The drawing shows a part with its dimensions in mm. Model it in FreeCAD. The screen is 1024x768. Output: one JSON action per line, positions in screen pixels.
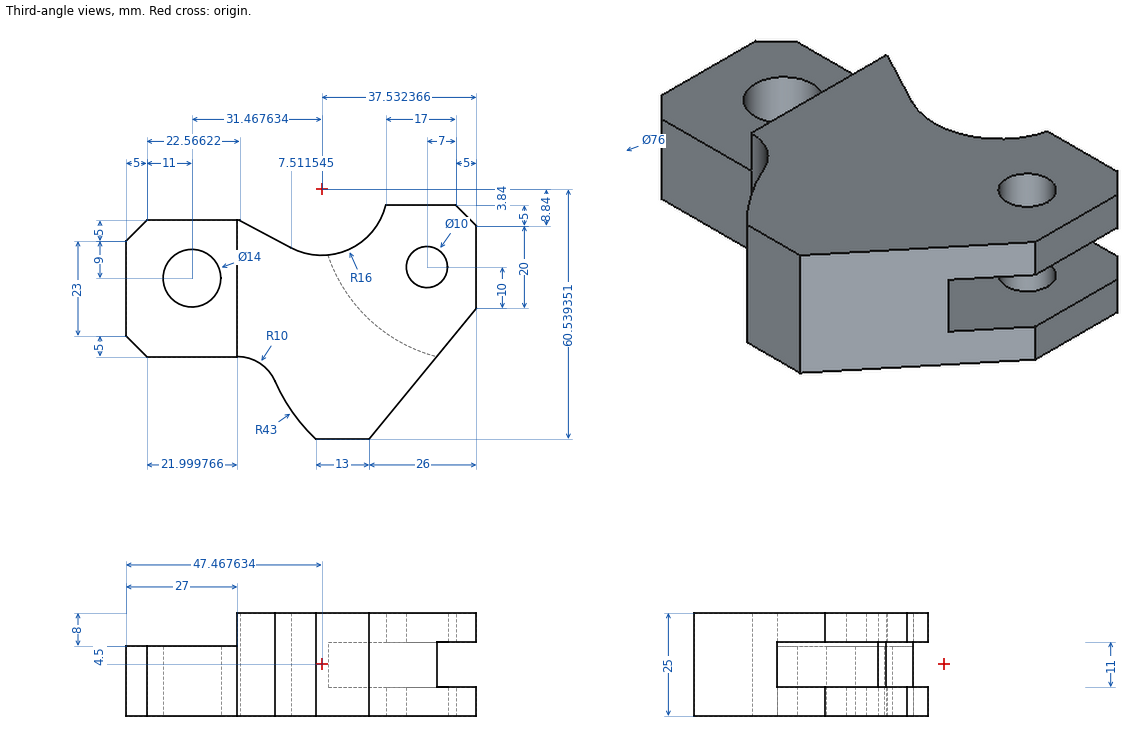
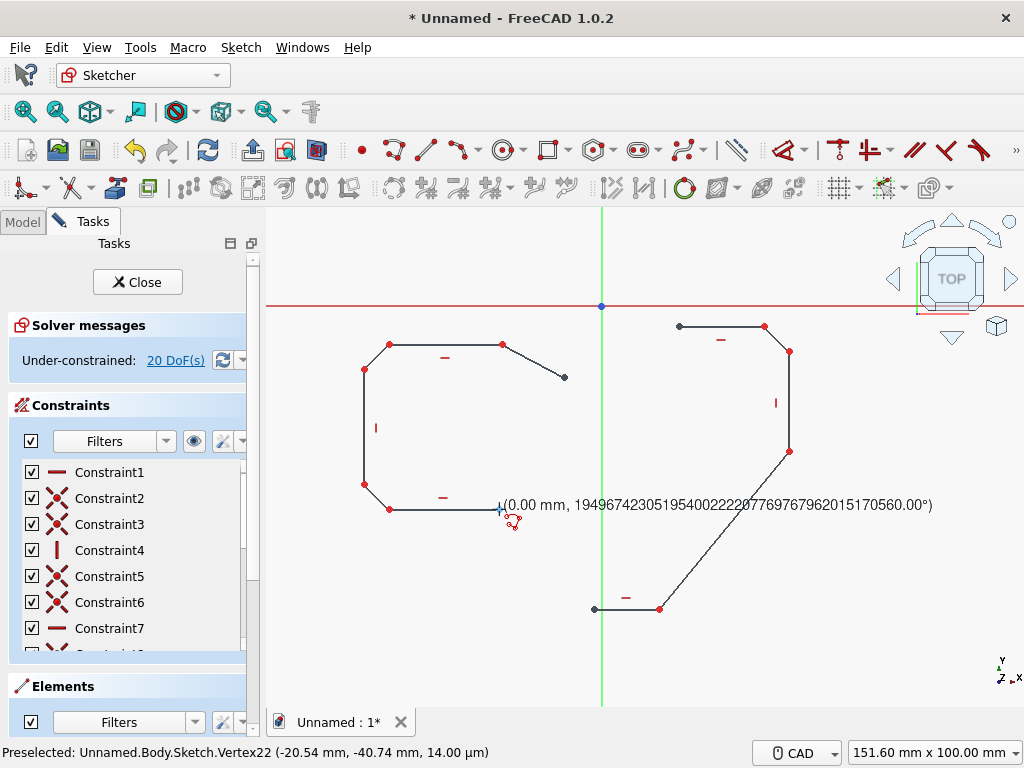
{"action": "left_click", "coordinate": [458, 150]}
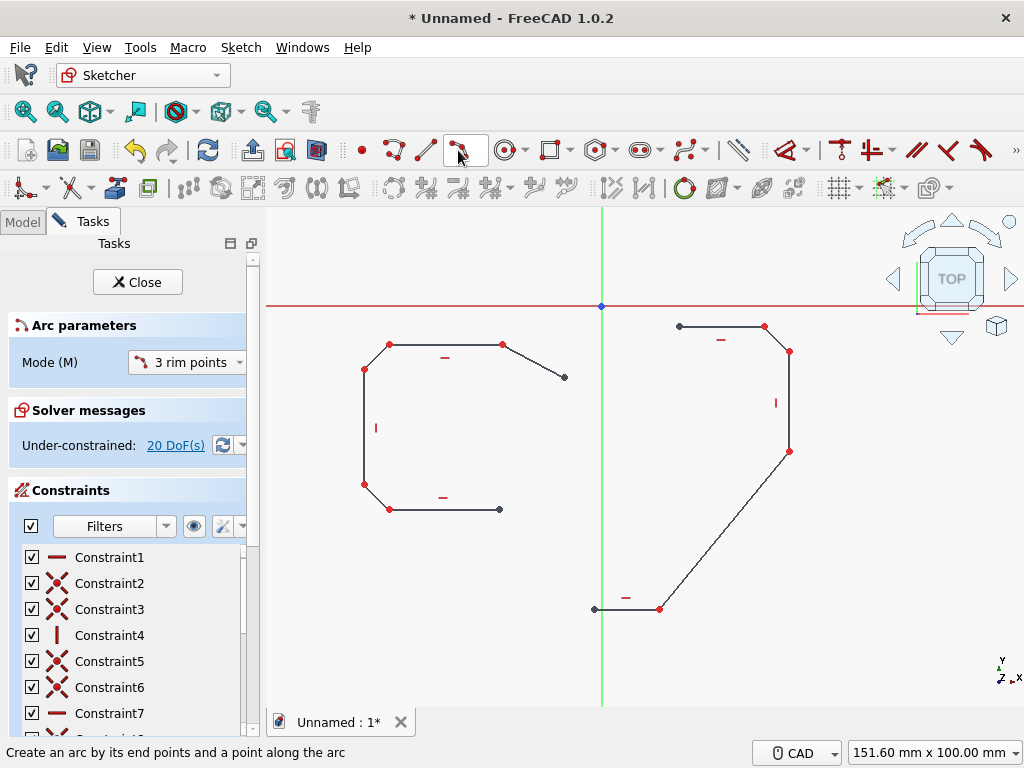
{"action": "left_click", "coordinate": [679, 327]}
{"action": "left_click", "coordinate": [564, 378]}
{"action": "left_click", "coordinate": [634, 379]}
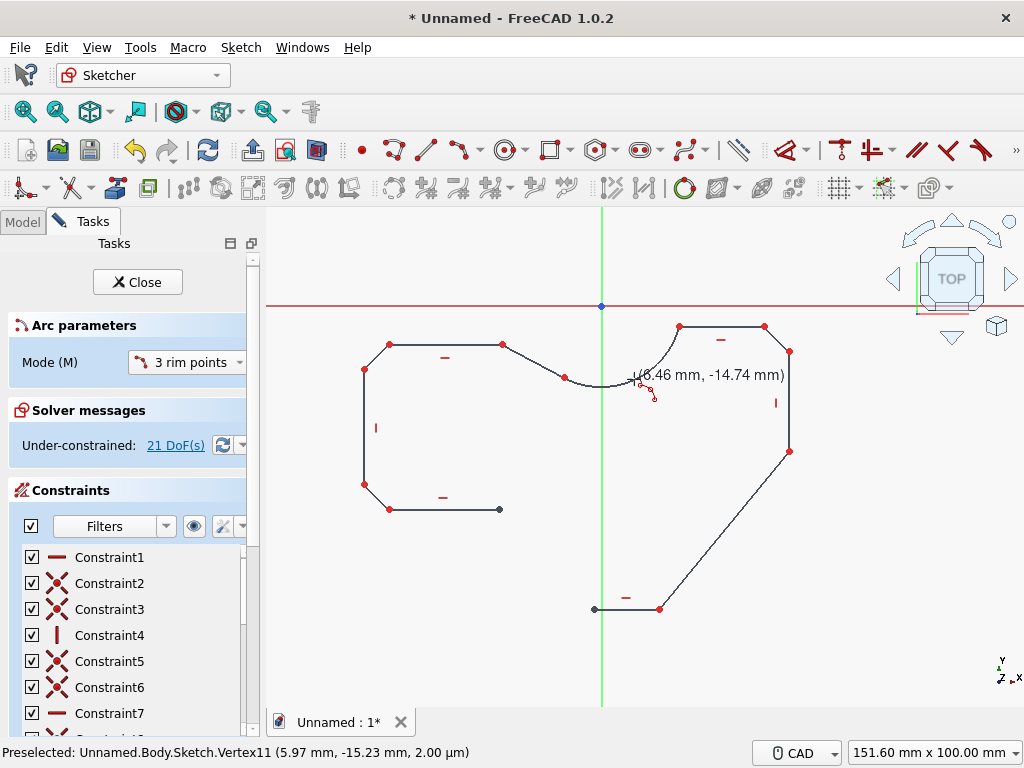
{"action": "left_click", "coordinate": [499, 510]}
{"action": "left_click", "coordinate": [545, 539]}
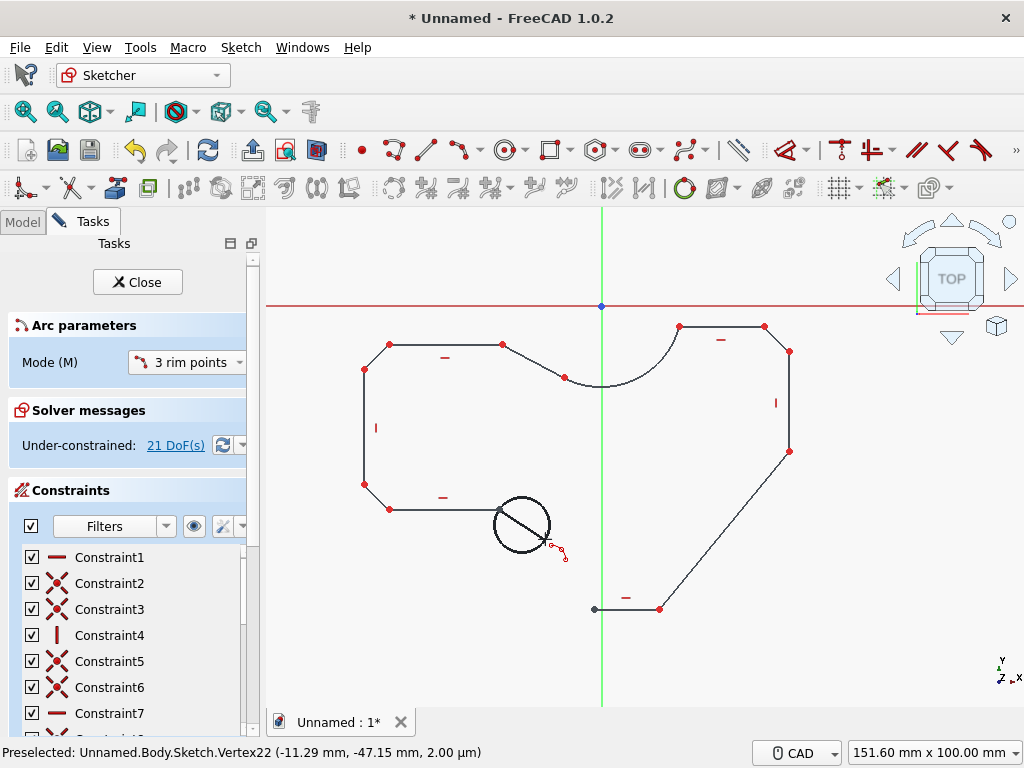
{"action": "scroll", "coordinate": [527, 517], "scroll_direction": "up", "scroll_amount": 4}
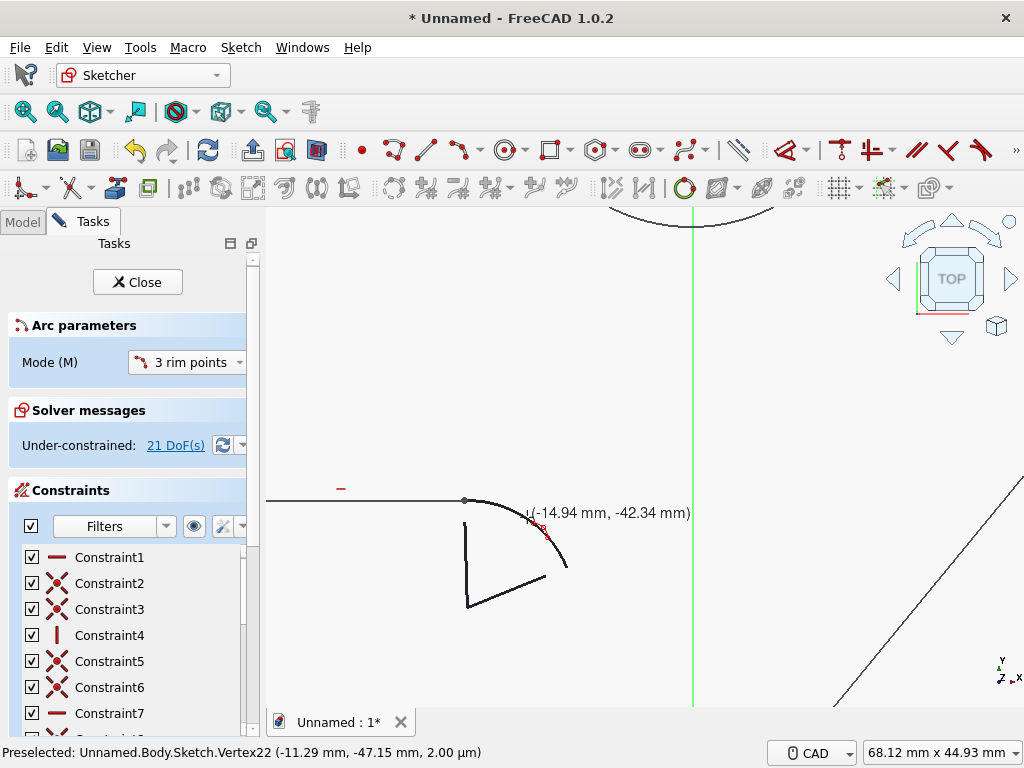
{"action": "left_click", "coordinate": [526, 517]}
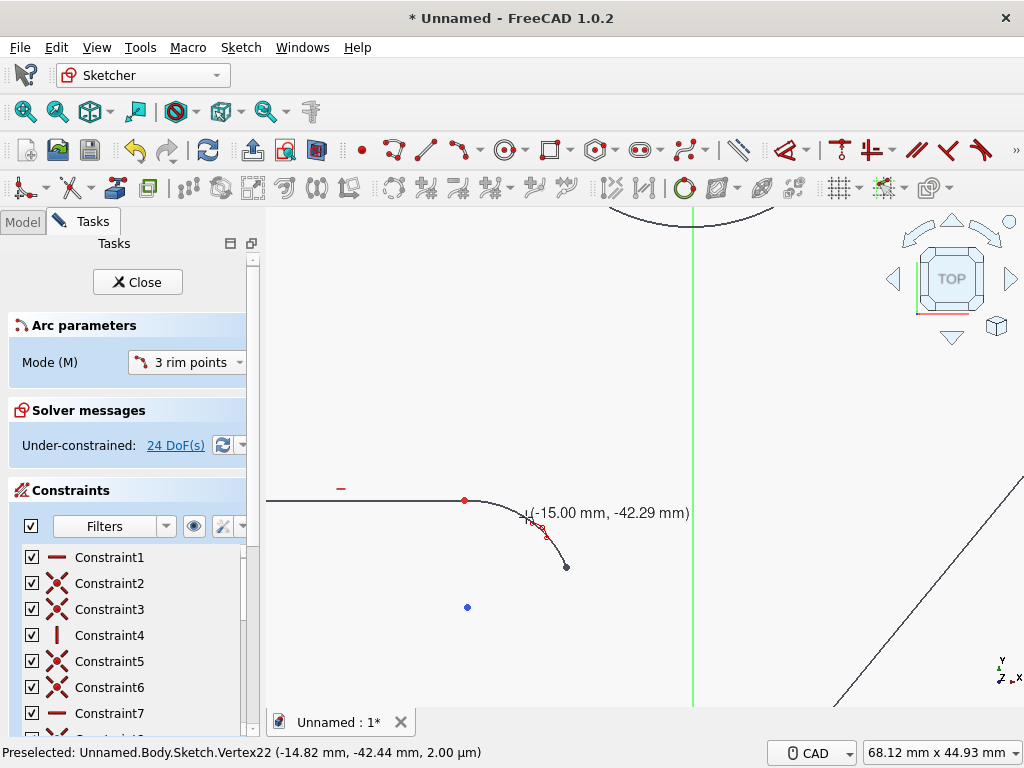
{"action": "left_click", "coordinate": [567, 567]}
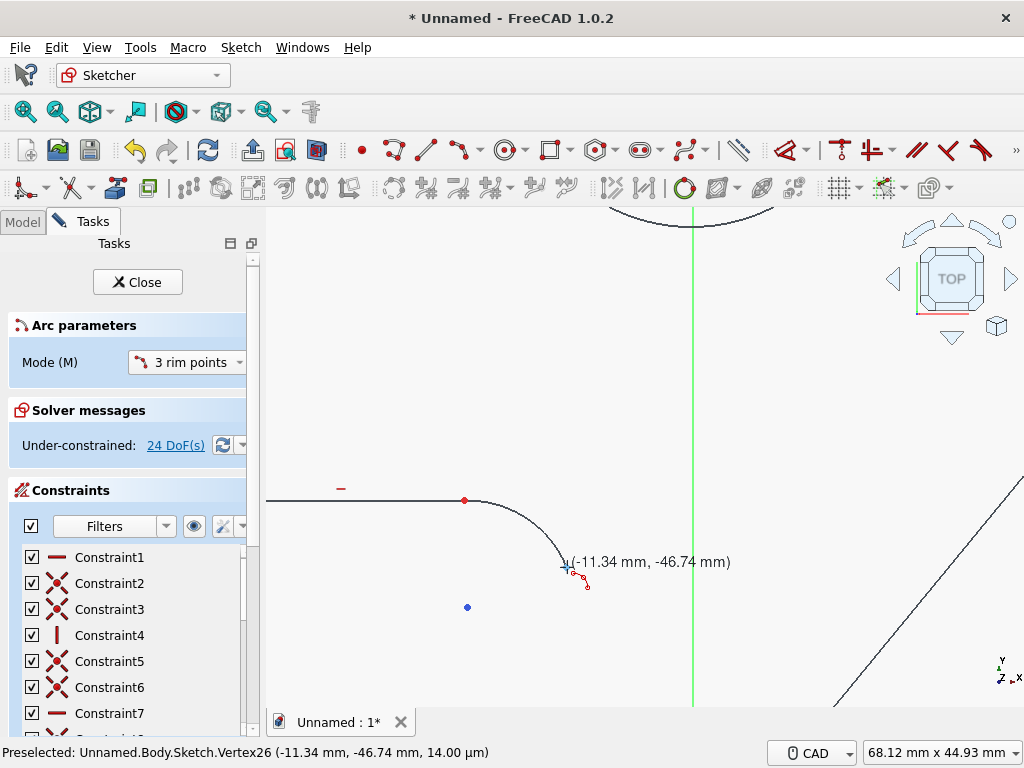
{"action": "scroll", "coordinate": [527, 516], "scroll_direction": "down", "scroll_amount": 4}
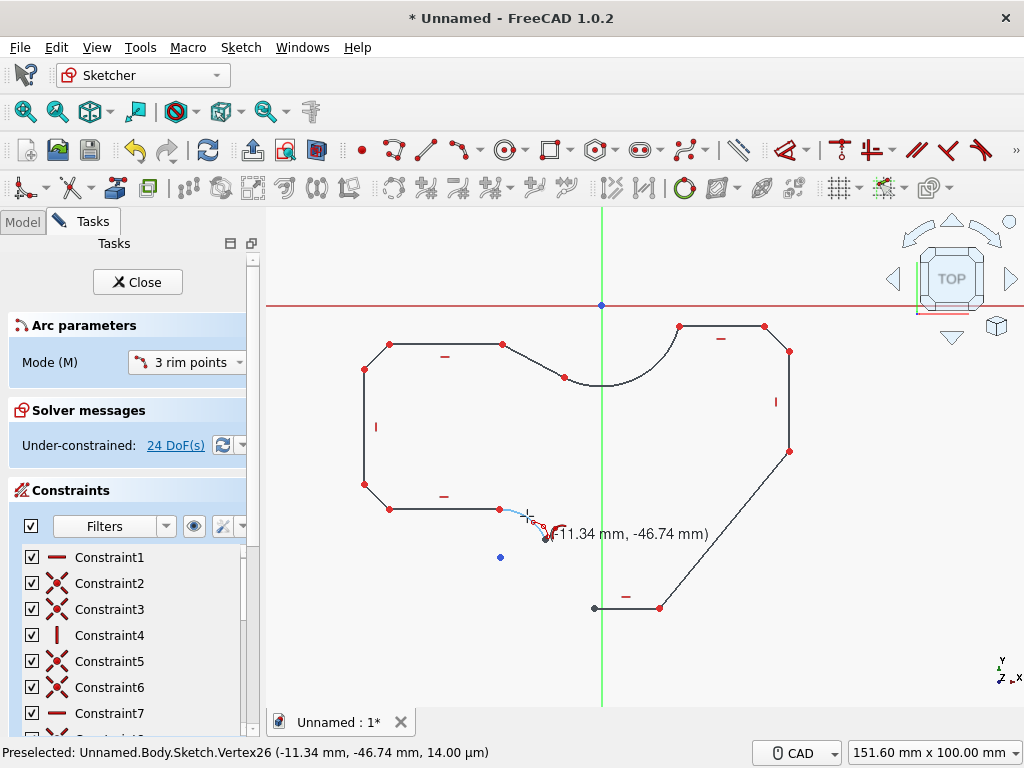
{"action": "scroll", "coordinate": [594, 608], "scroll_direction": "up", "scroll_amount": 4}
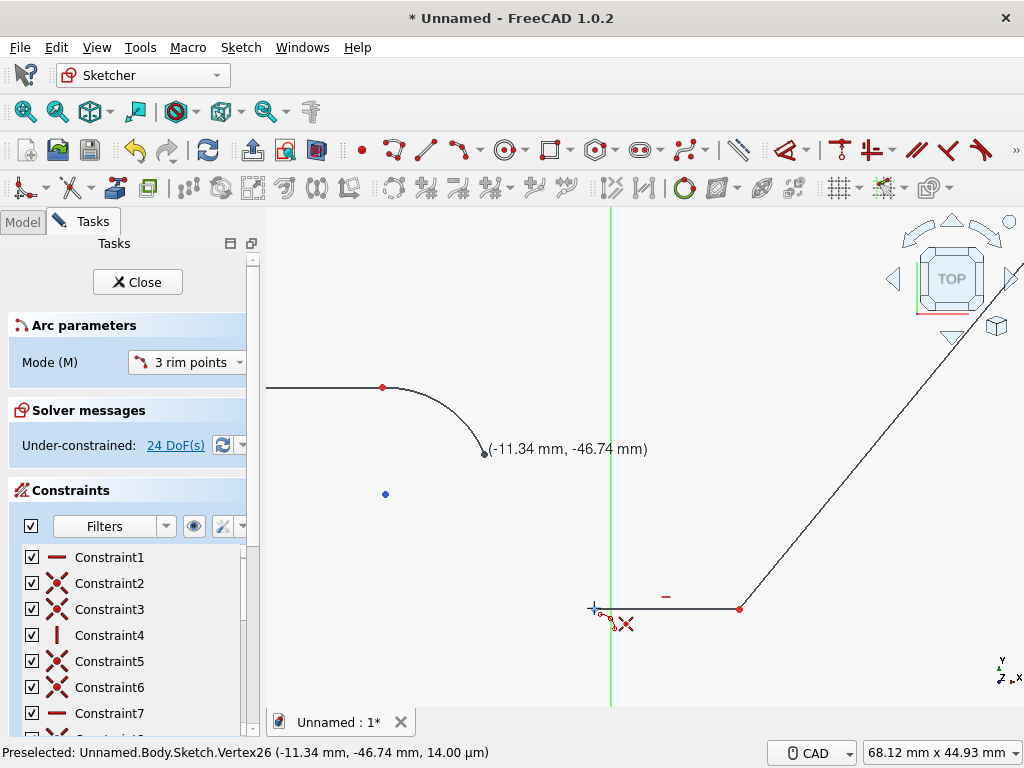
{"action": "left_click", "coordinate": [594, 609]}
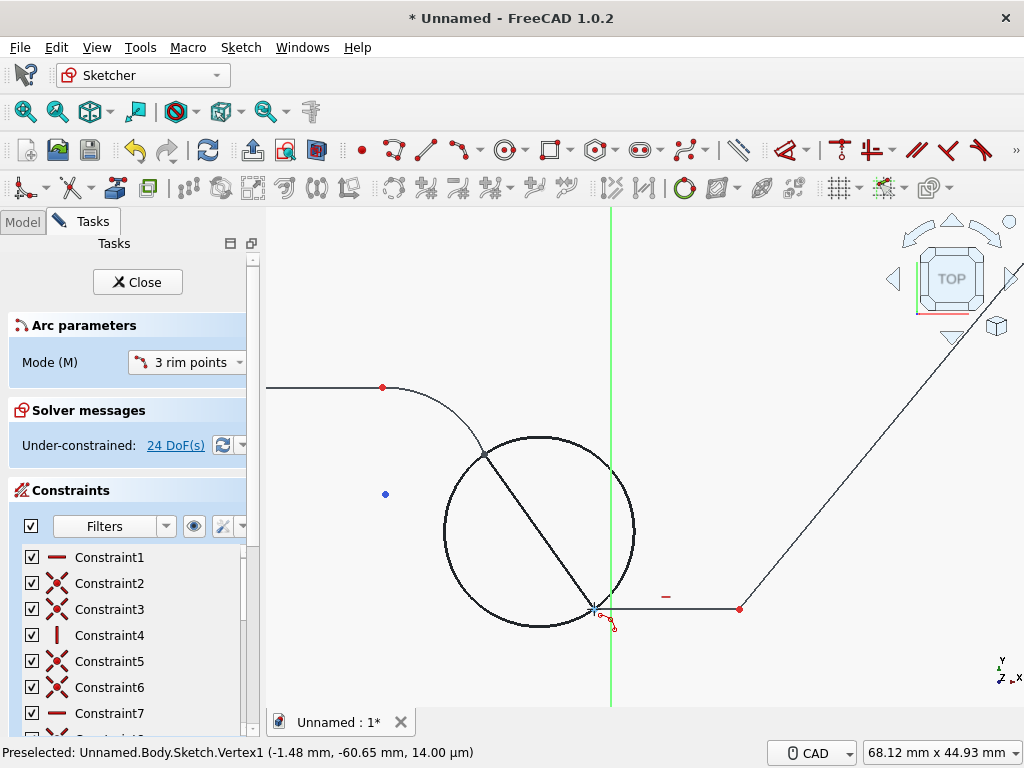
{"action": "scroll", "coordinate": [532, 536], "scroll_direction": "up", "scroll_amount": 3}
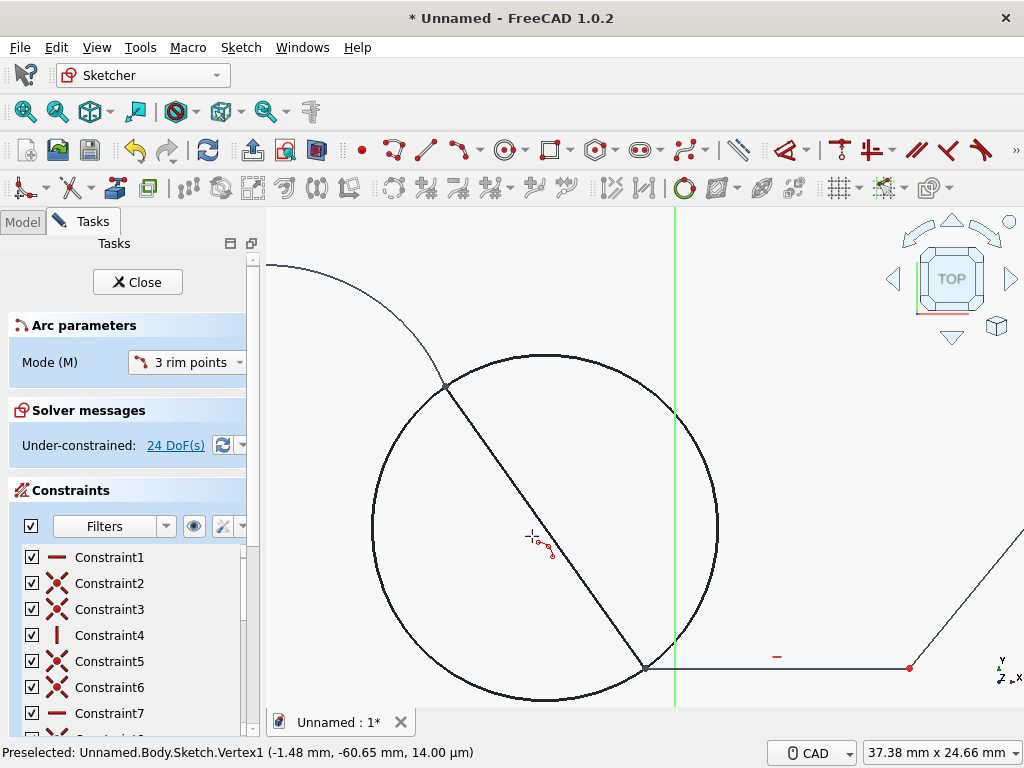
{"action": "left_click", "coordinate": [531, 535]}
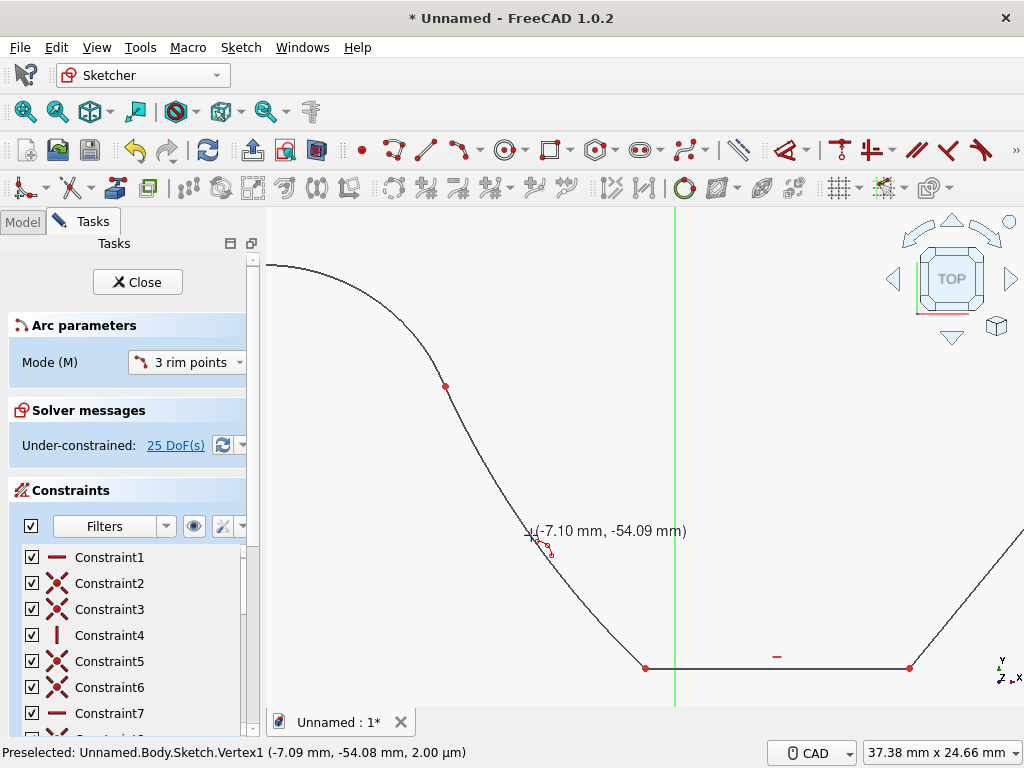
{"action": "left_click", "coordinate": [506, 150]}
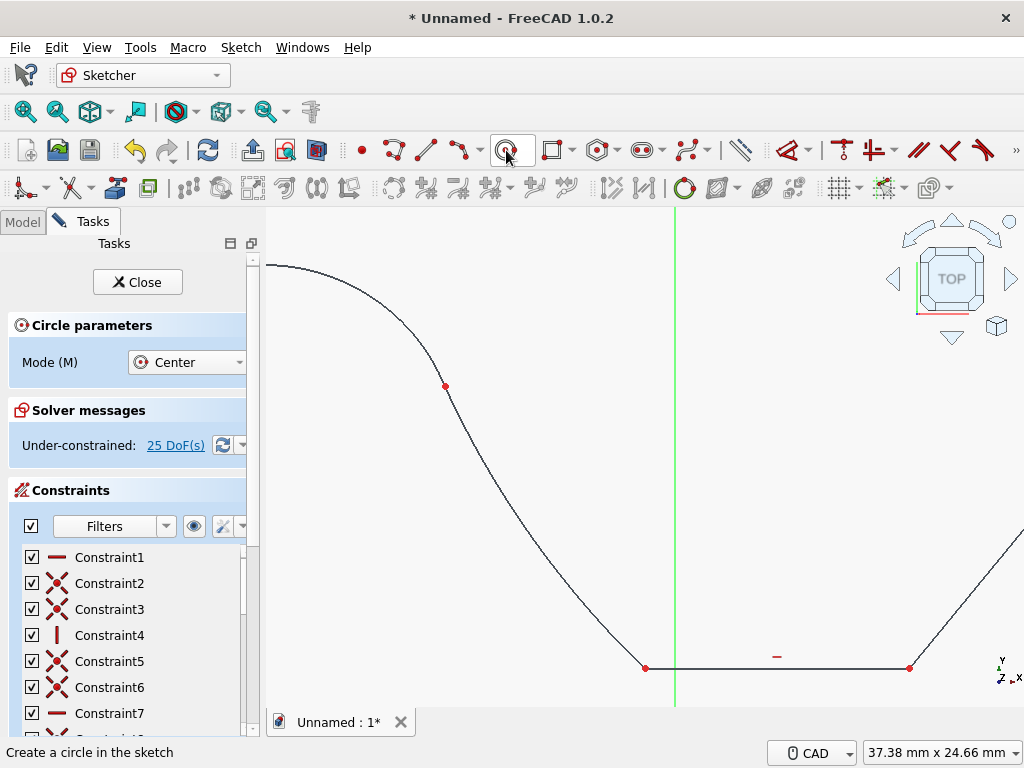
{"action": "scroll", "coordinate": [577, 589], "scroll_direction": "down", "scroll_amount": 7}